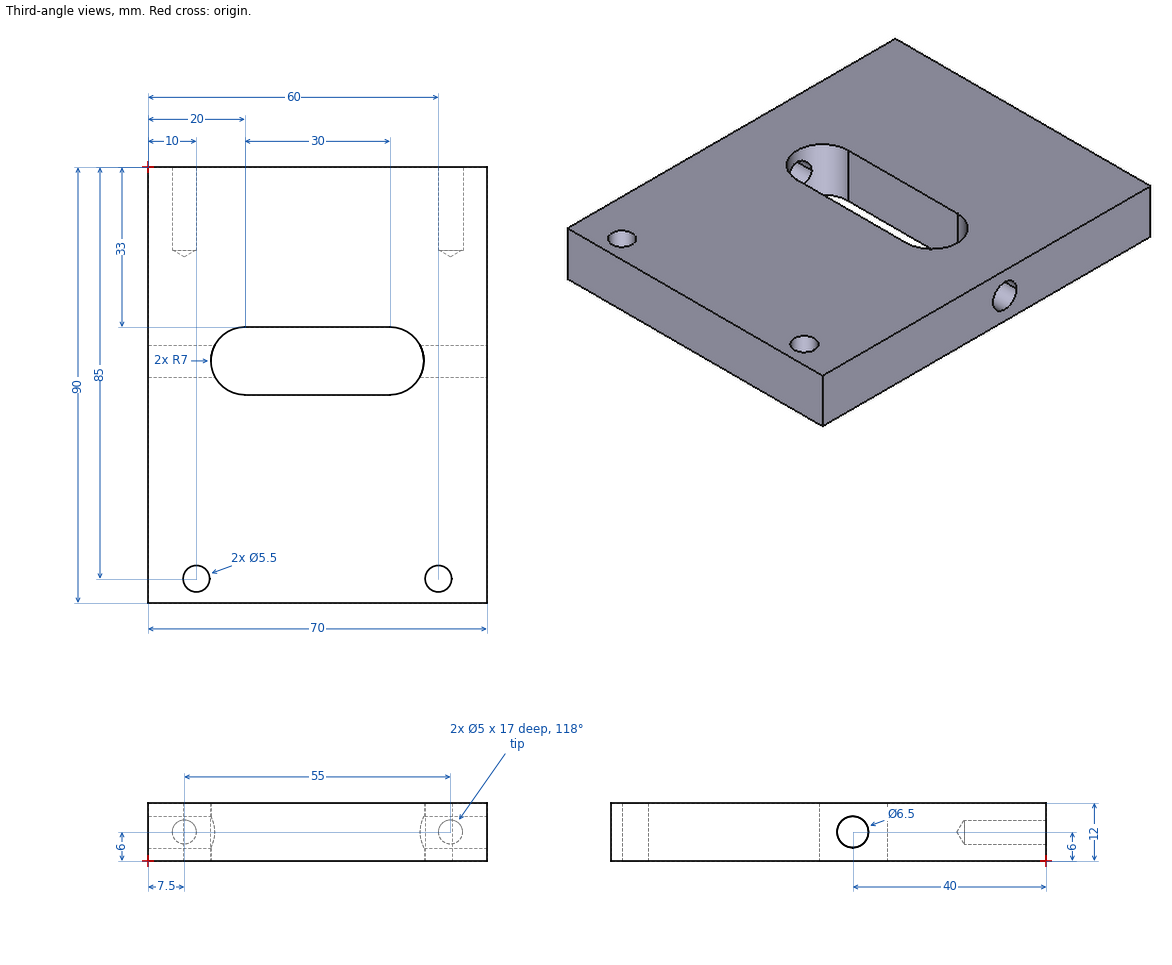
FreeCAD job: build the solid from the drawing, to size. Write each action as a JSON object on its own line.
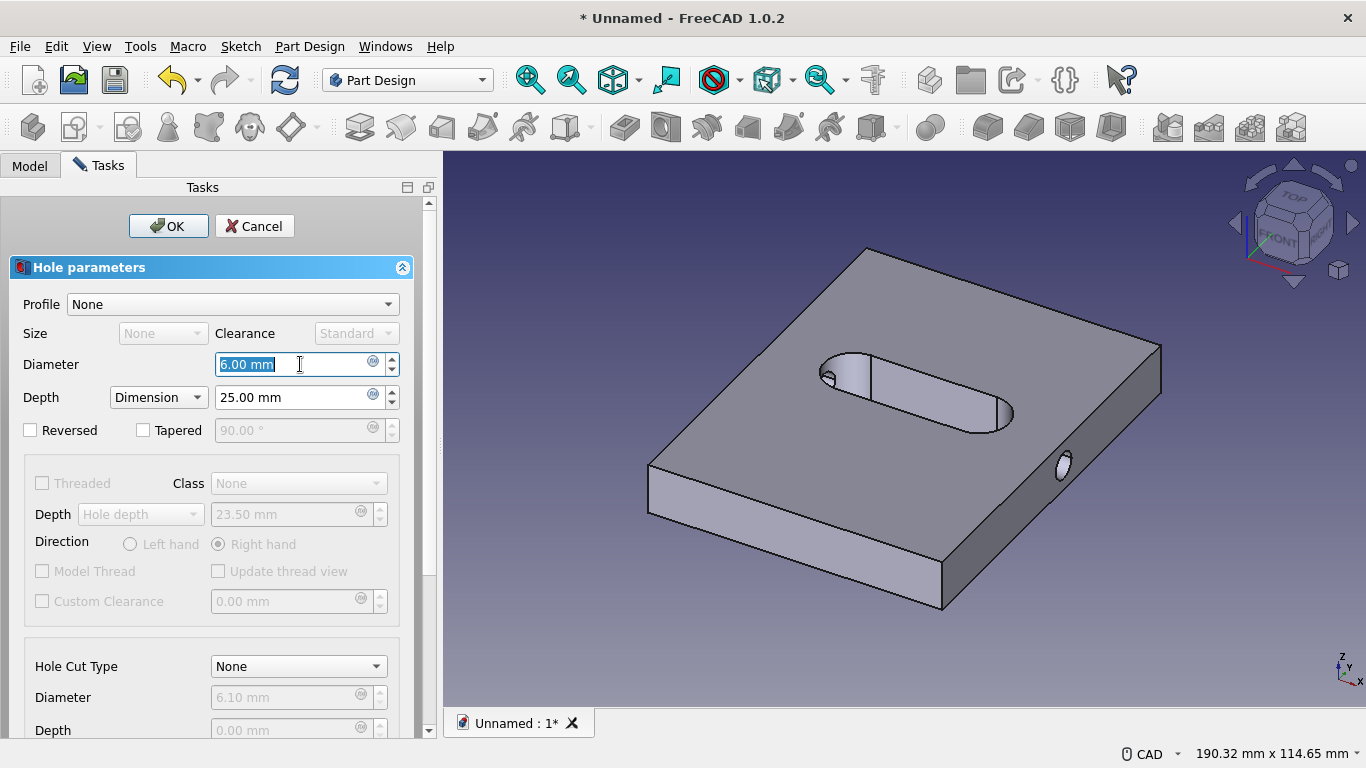
{"action": "type", "text": "5"}
{"action": "key", "text": "Tab"}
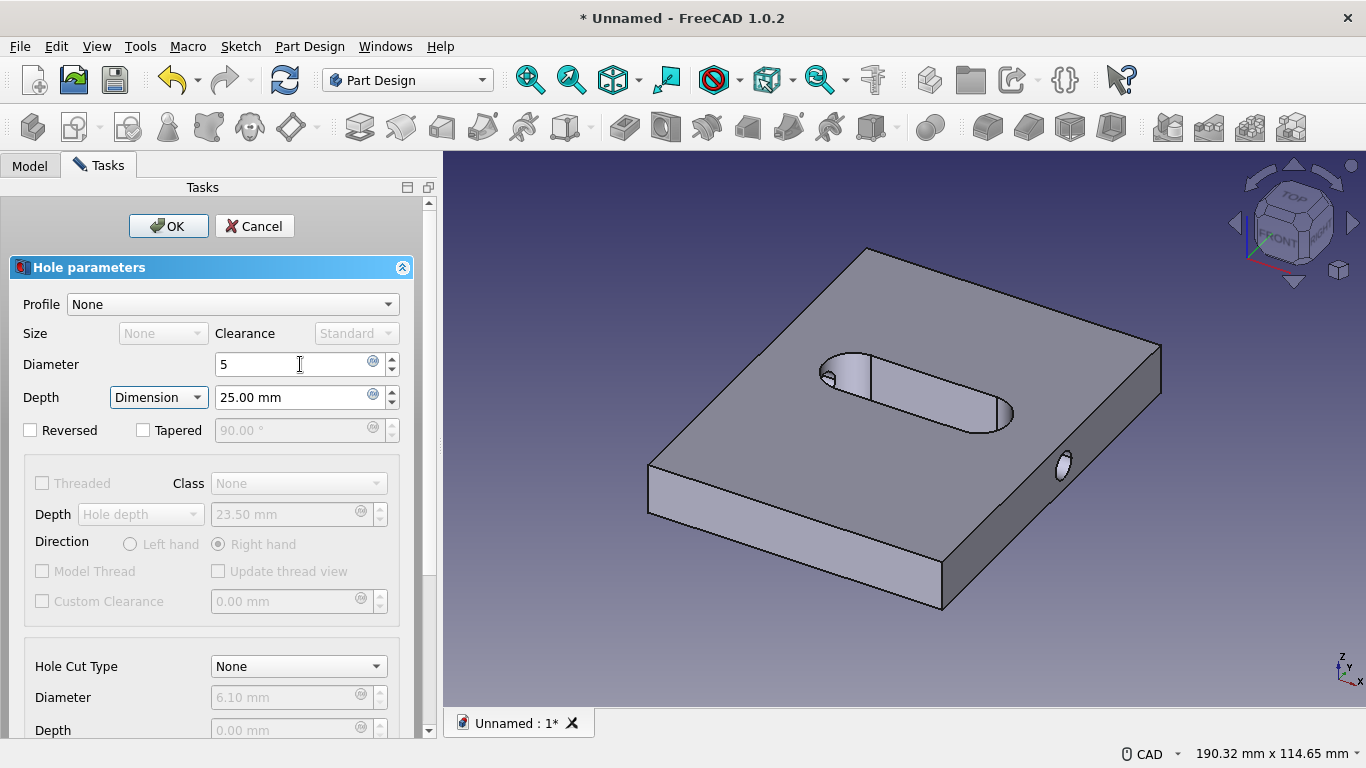
{"action": "triple_click", "coordinate": [300, 398]}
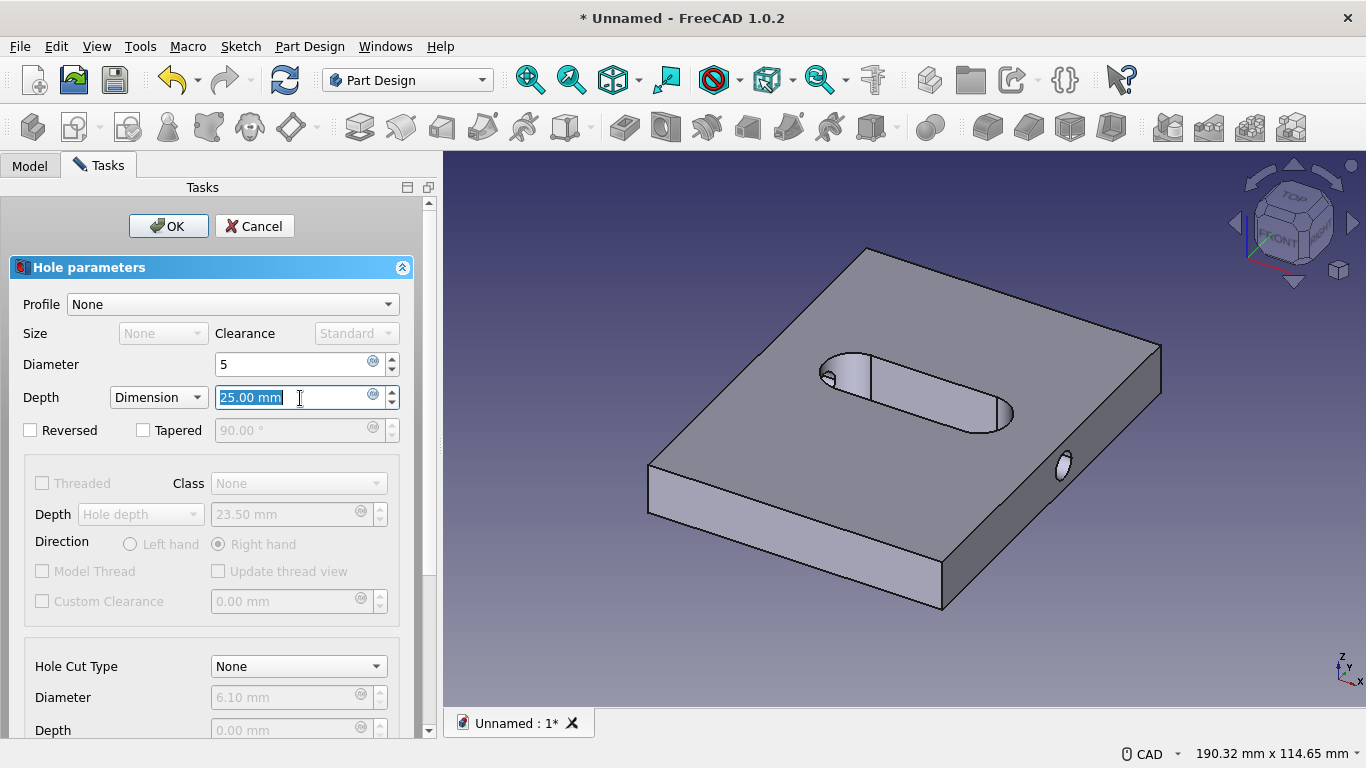
{"action": "type", "text": "17"}
{"action": "key", "text": "Tab"}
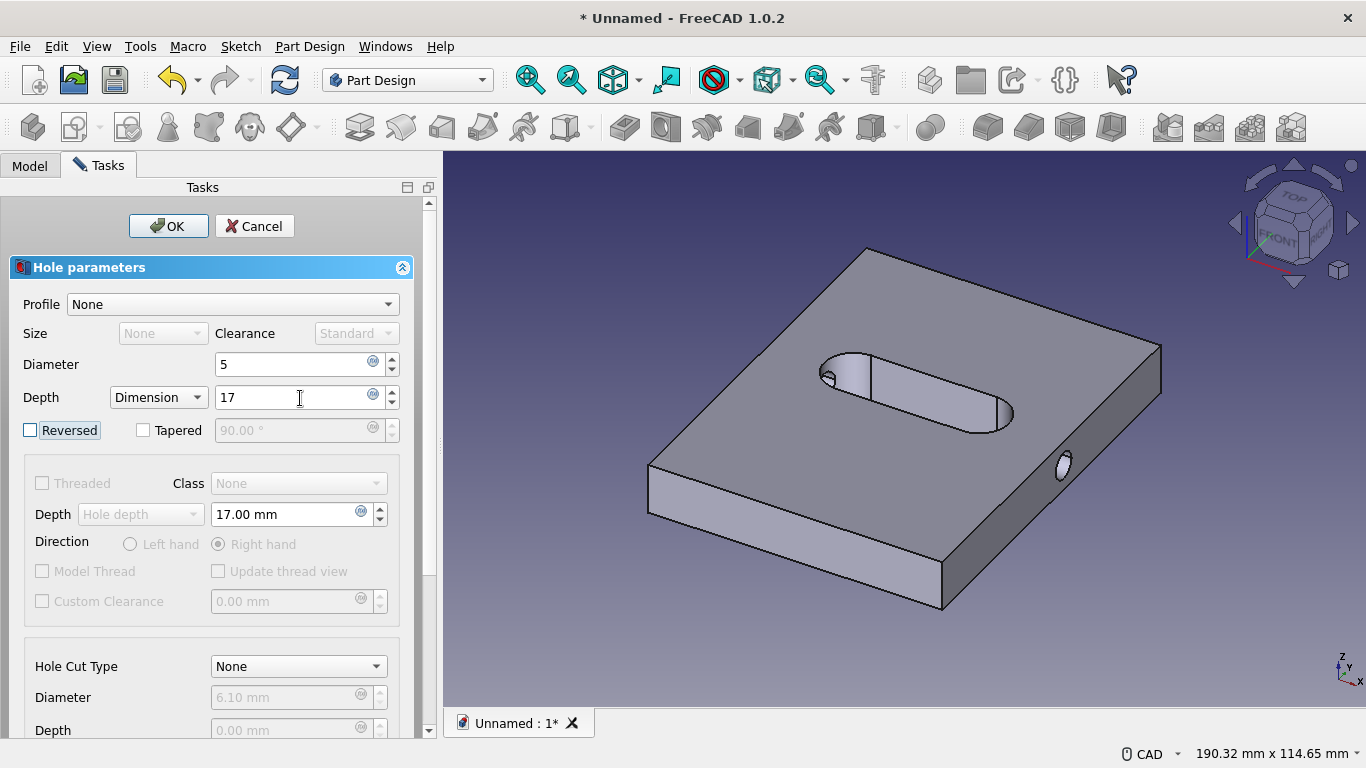
{"action": "left_click", "coordinate": [31, 430]}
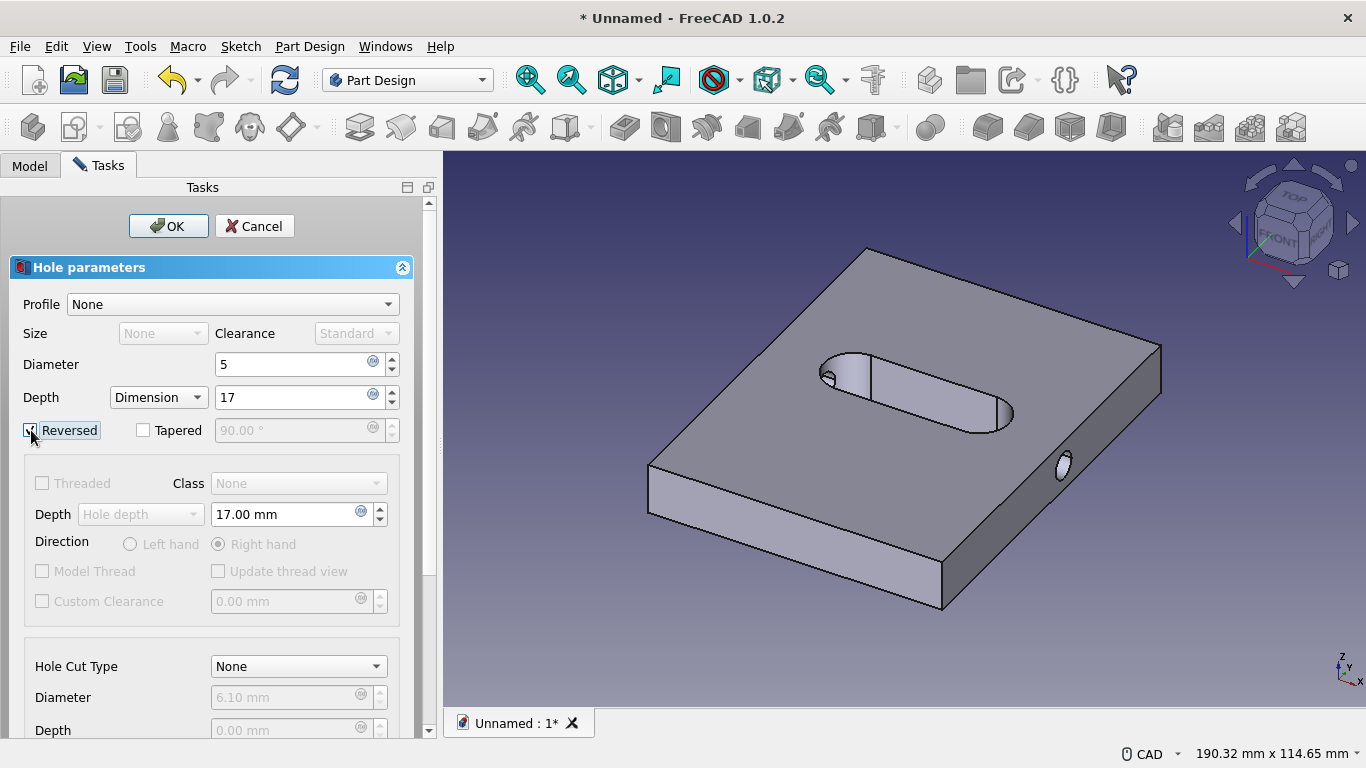
{"action": "left_click", "coordinate": [169, 226]}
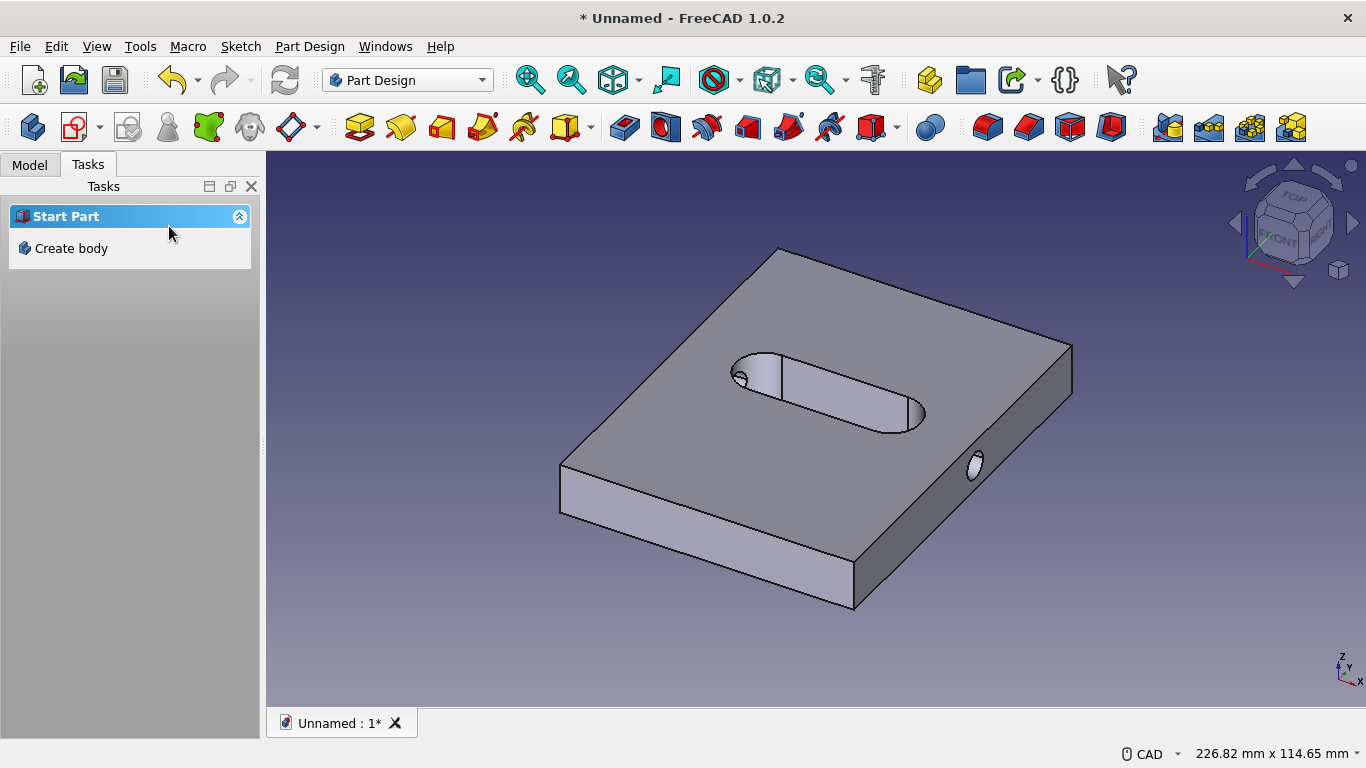
{"action": "left_click", "coordinate": [796, 480]}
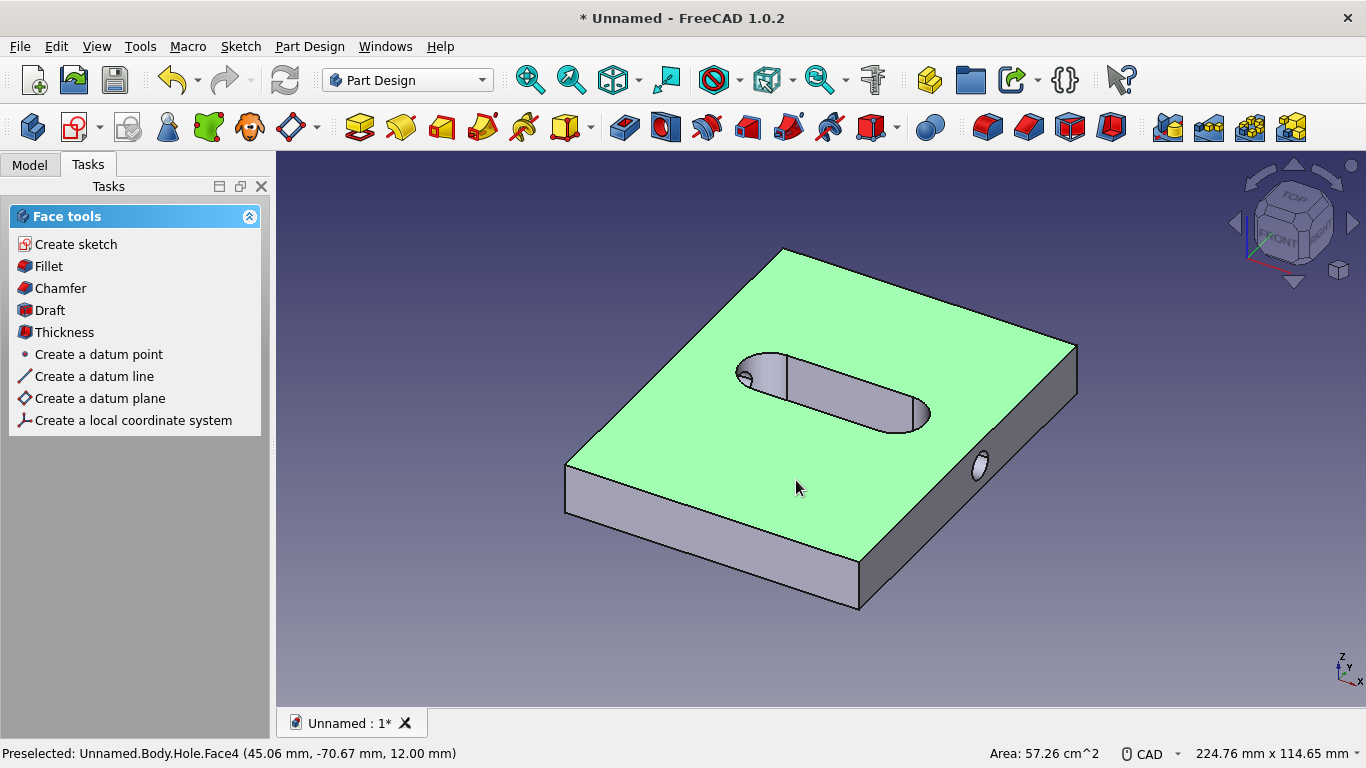
{"action": "left_click", "coordinate": [74, 128]}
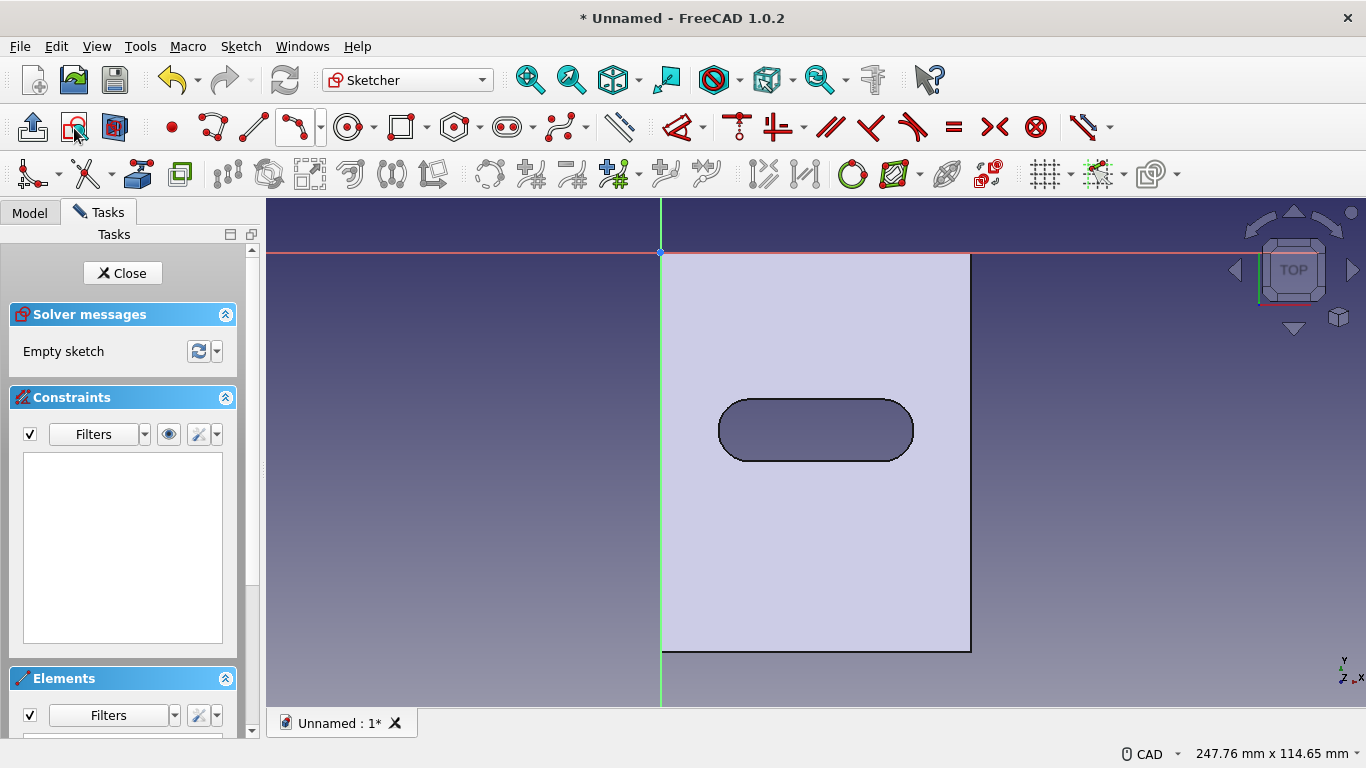
{"action": "left_click", "coordinate": [348, 128]}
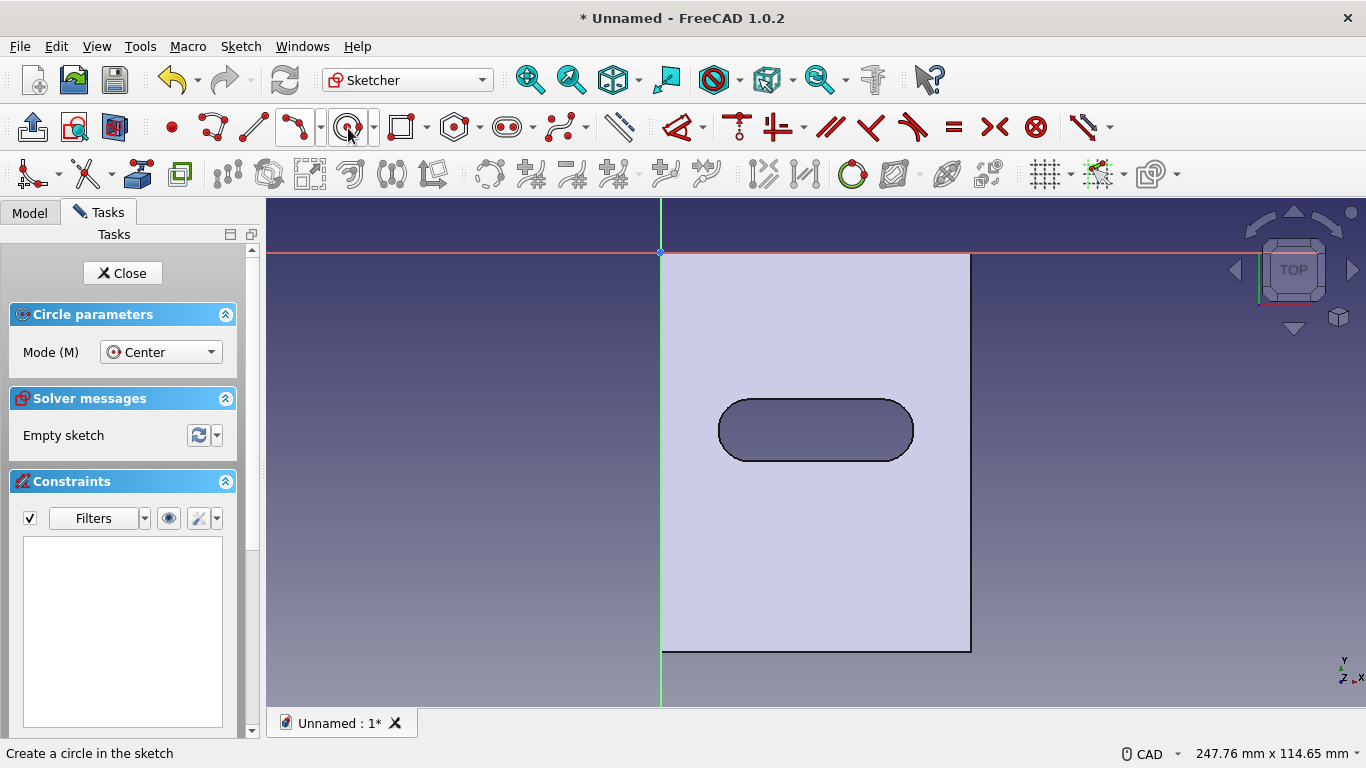
{"action": "scroll", "coordinate": [705, 630], "scroll_direction": "up", "scroll_amount": 4}